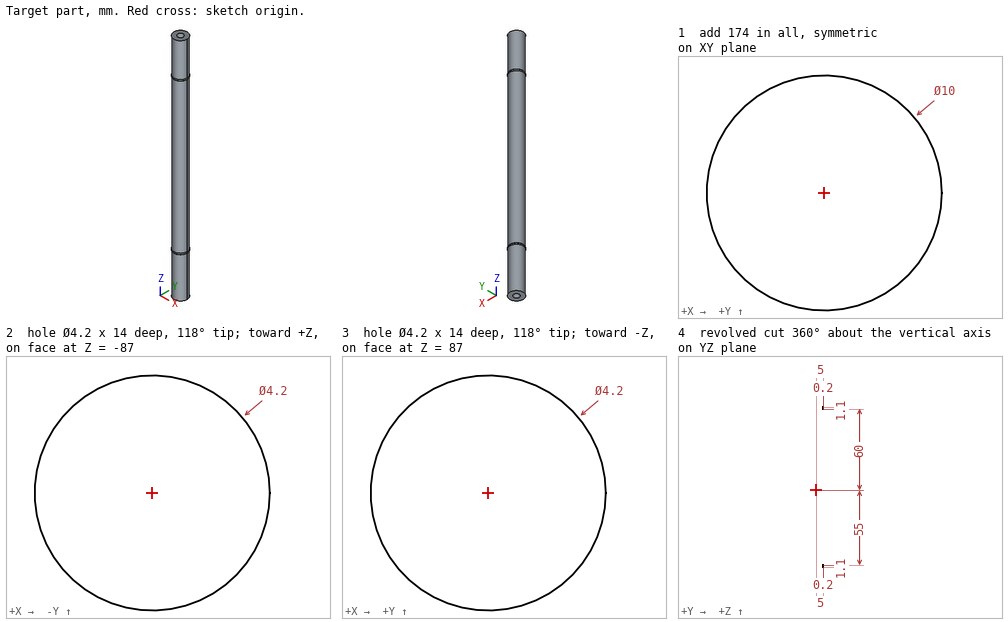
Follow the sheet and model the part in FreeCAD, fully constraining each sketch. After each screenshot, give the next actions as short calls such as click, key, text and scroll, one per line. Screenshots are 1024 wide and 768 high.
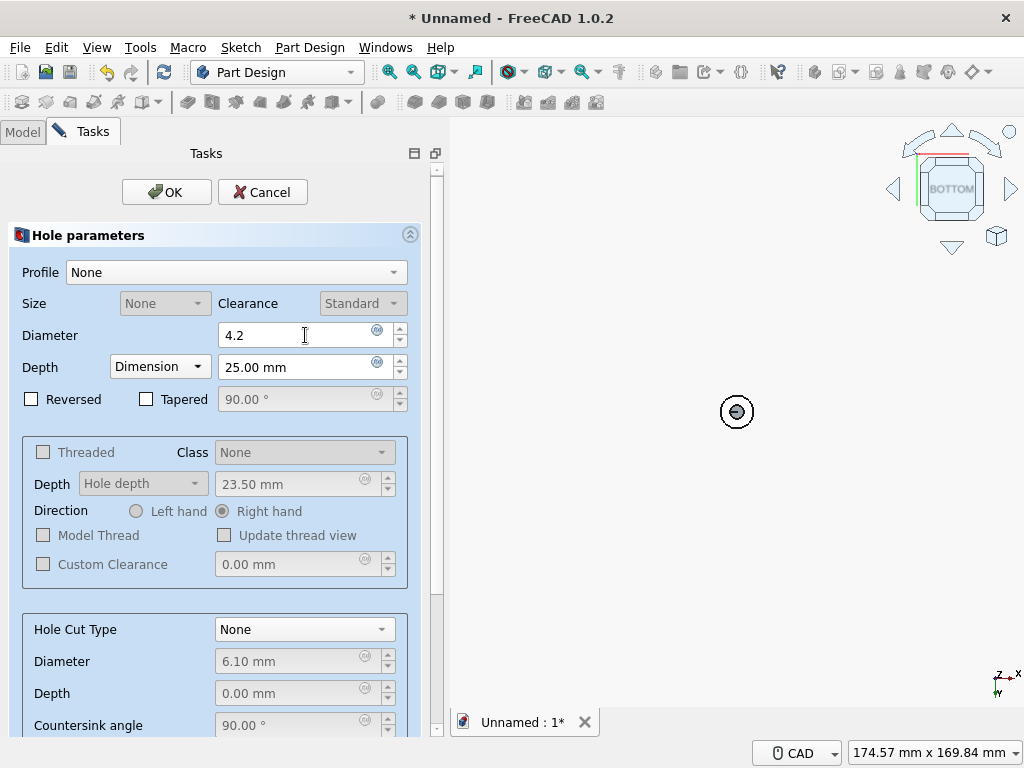
triple_click(305, 367)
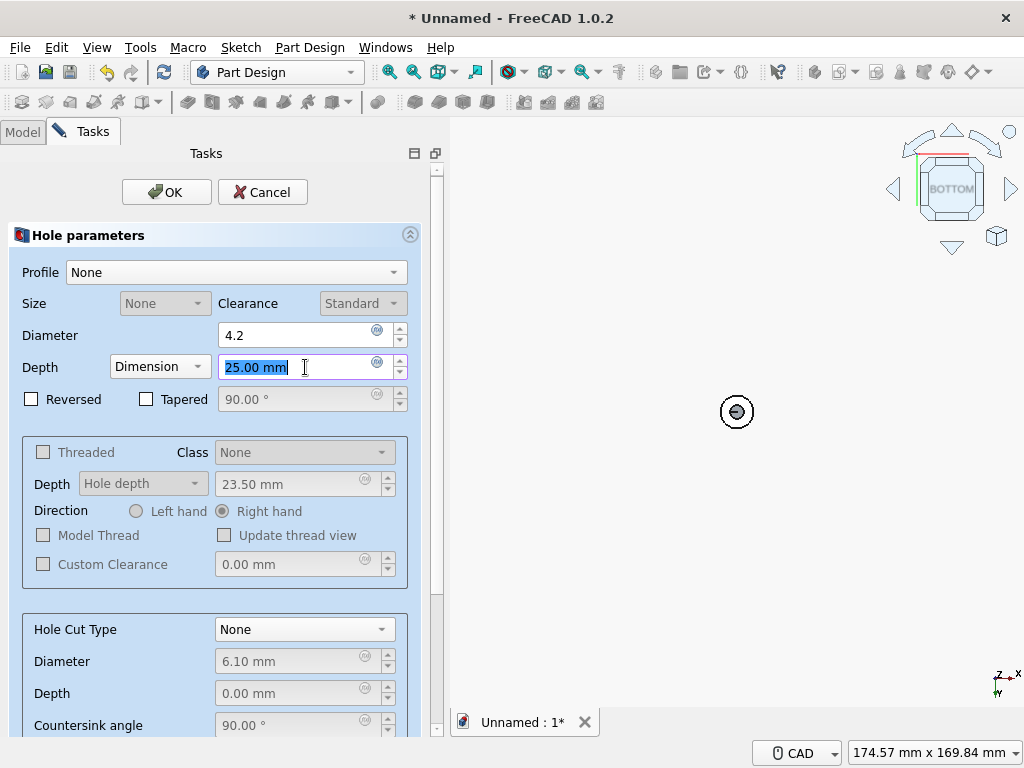
text(14)
key(Tab)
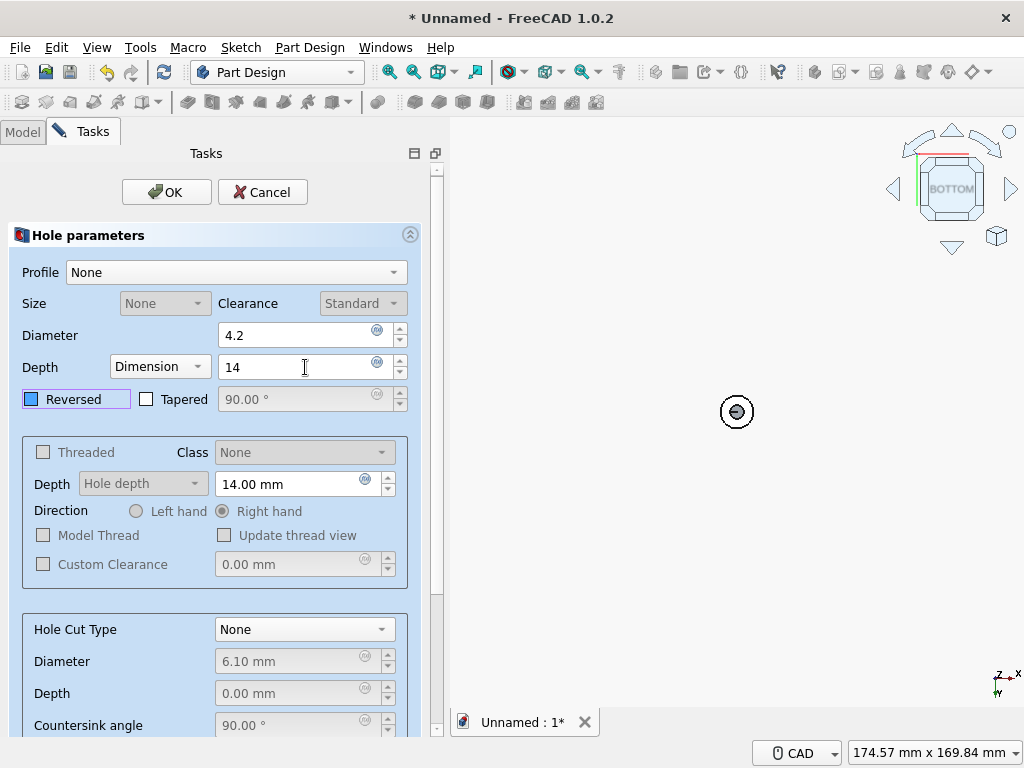
click(167, 192)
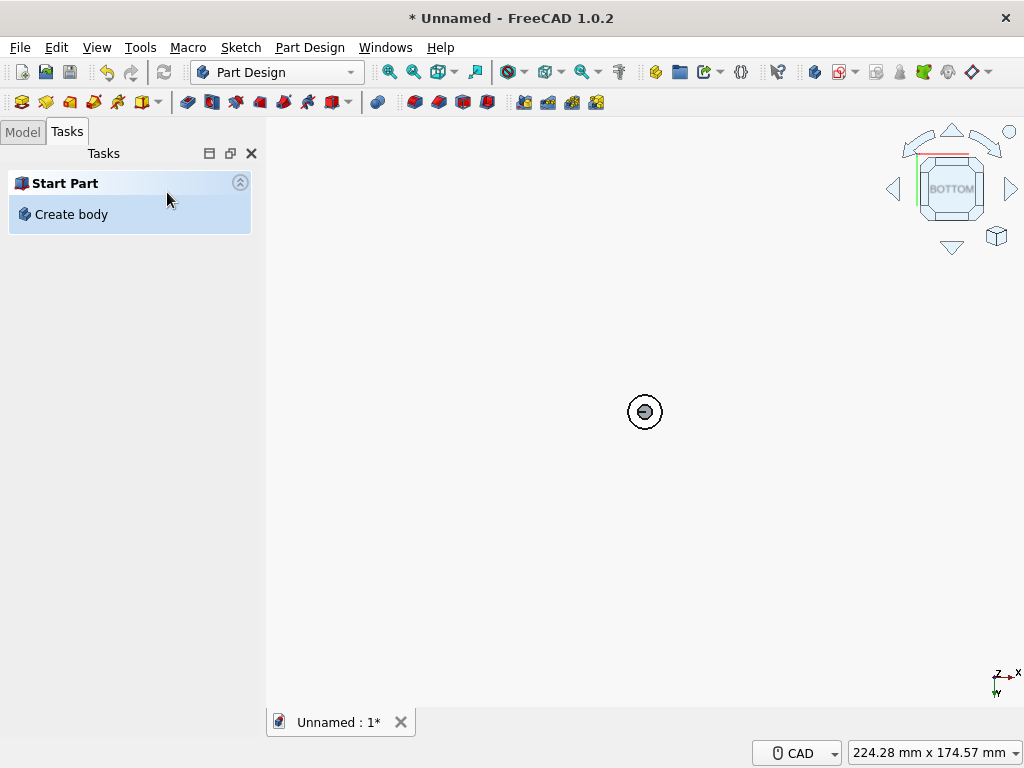
click(390, 72)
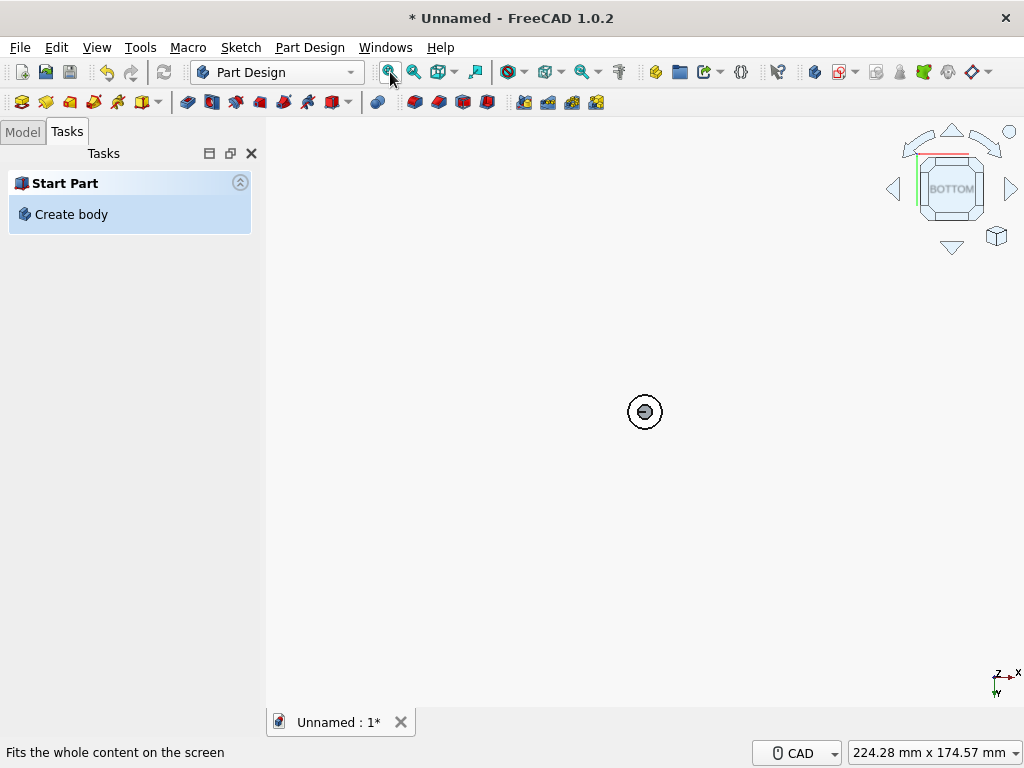
key(0)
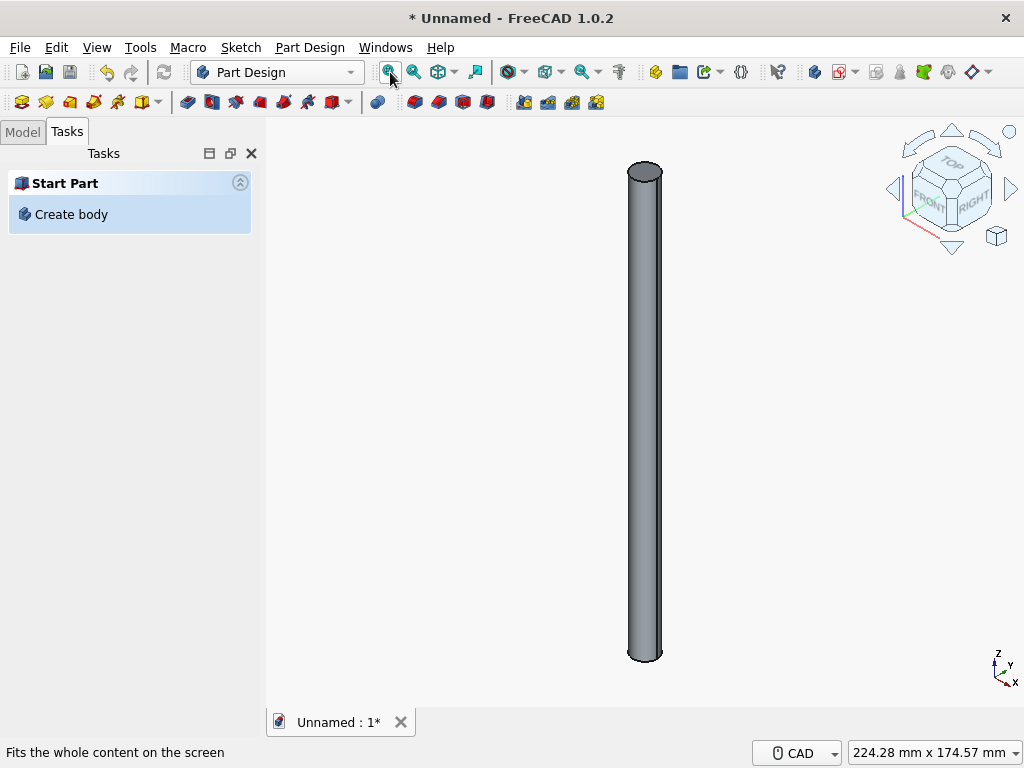
click(645, 171)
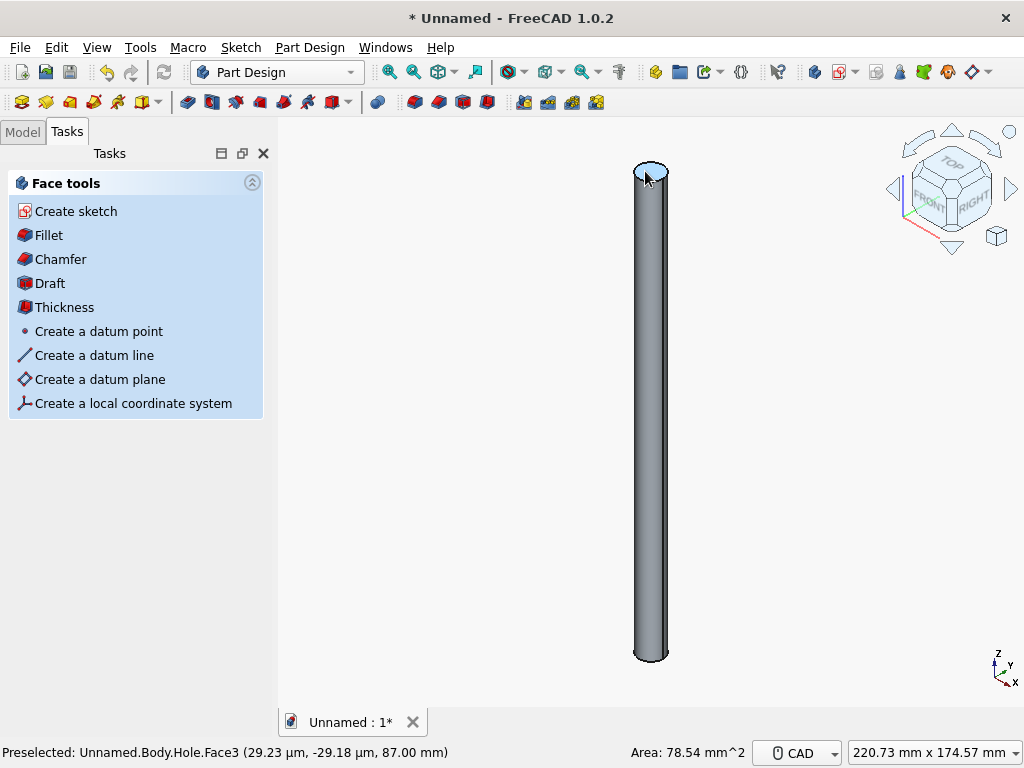
click(840, 72)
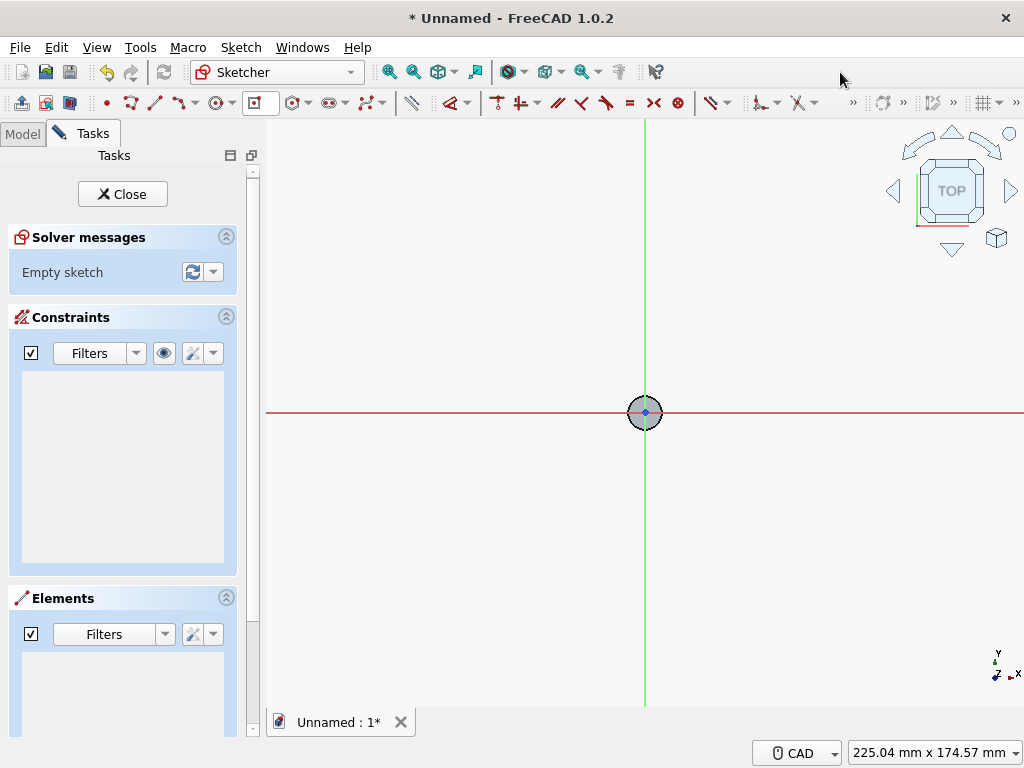
scroll(649, 413, up, 15)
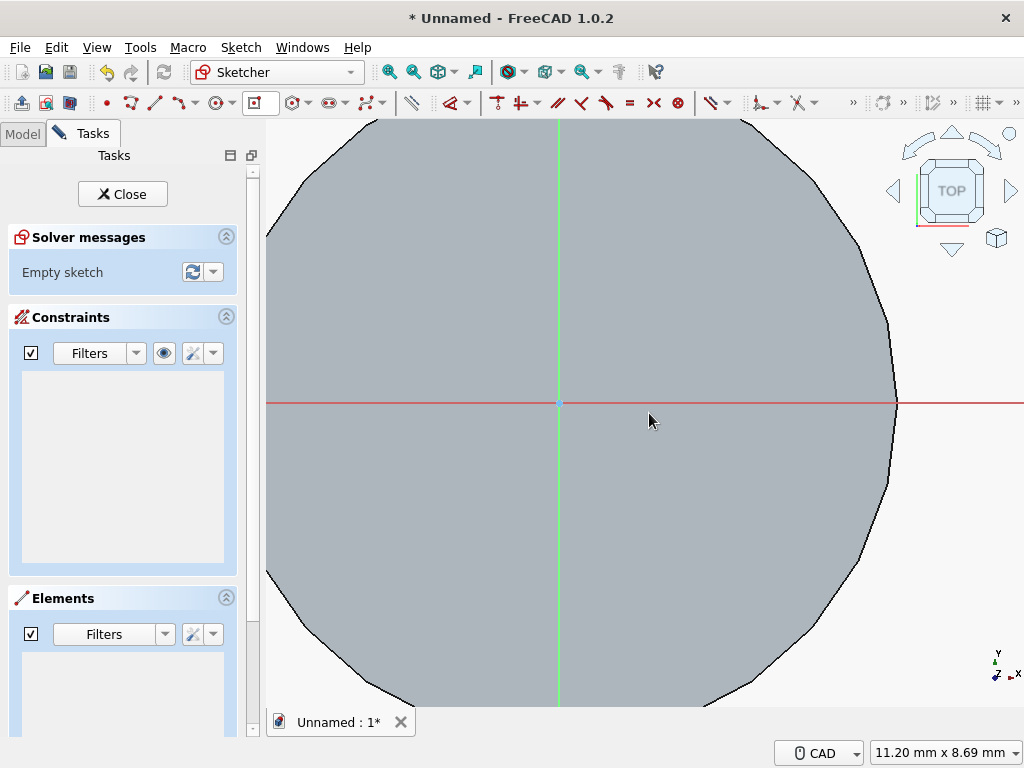
click(216, 104)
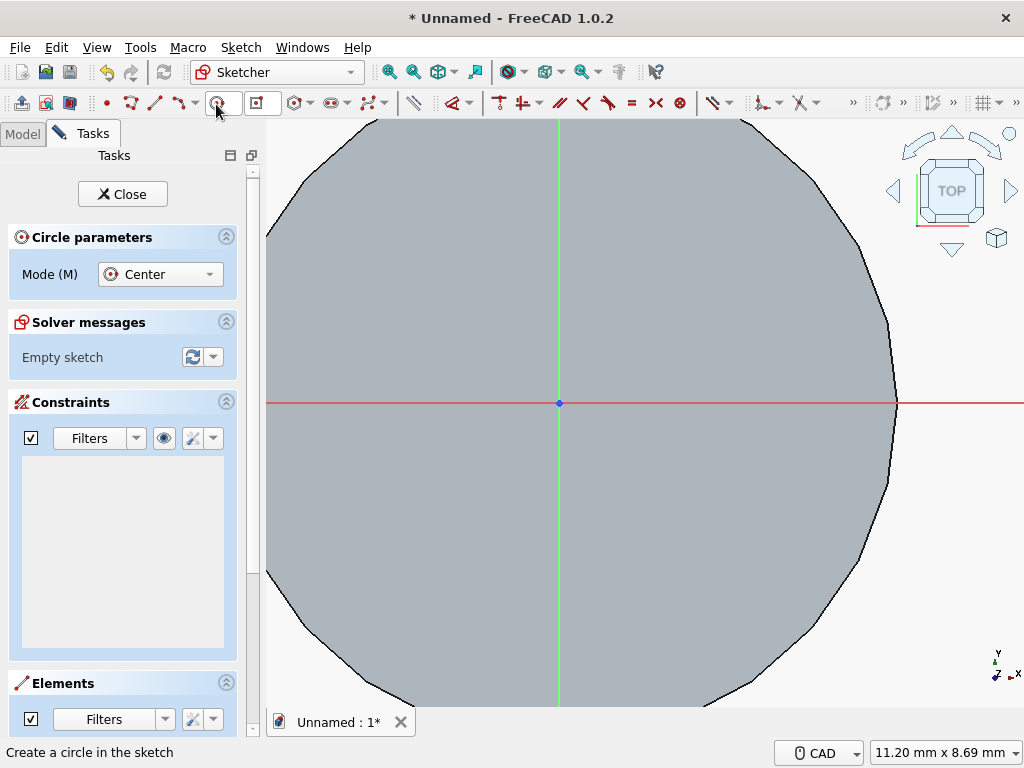
click(559, 403)
move(659, 303)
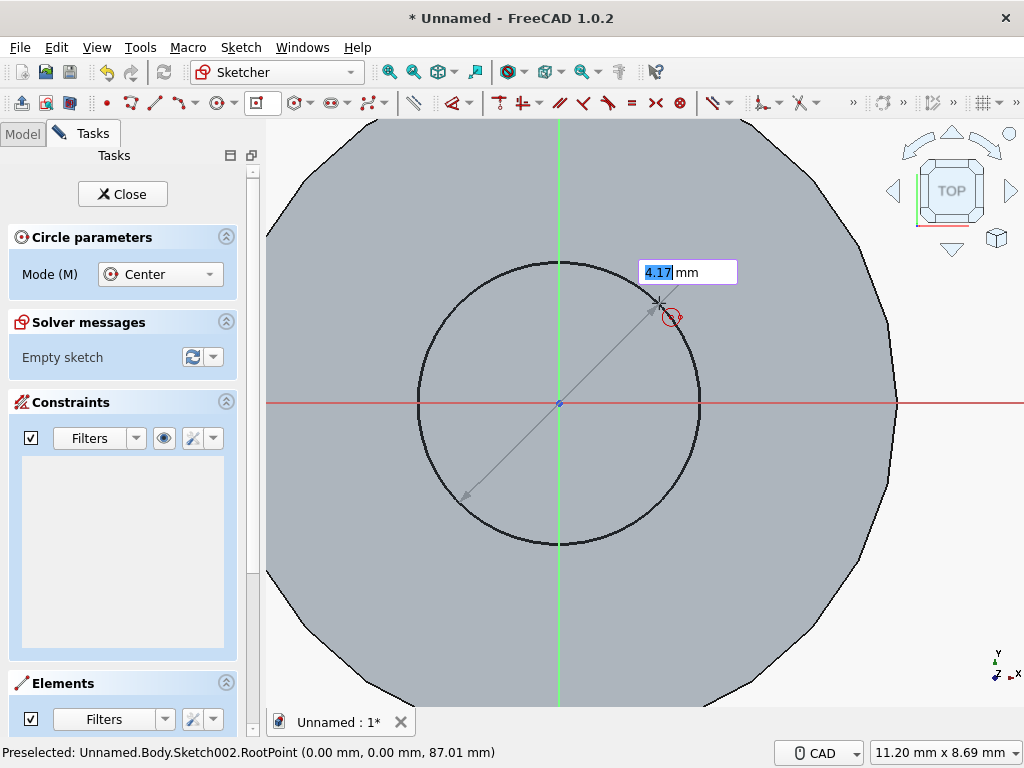
text(4.2)
key(Return)
key(Escape)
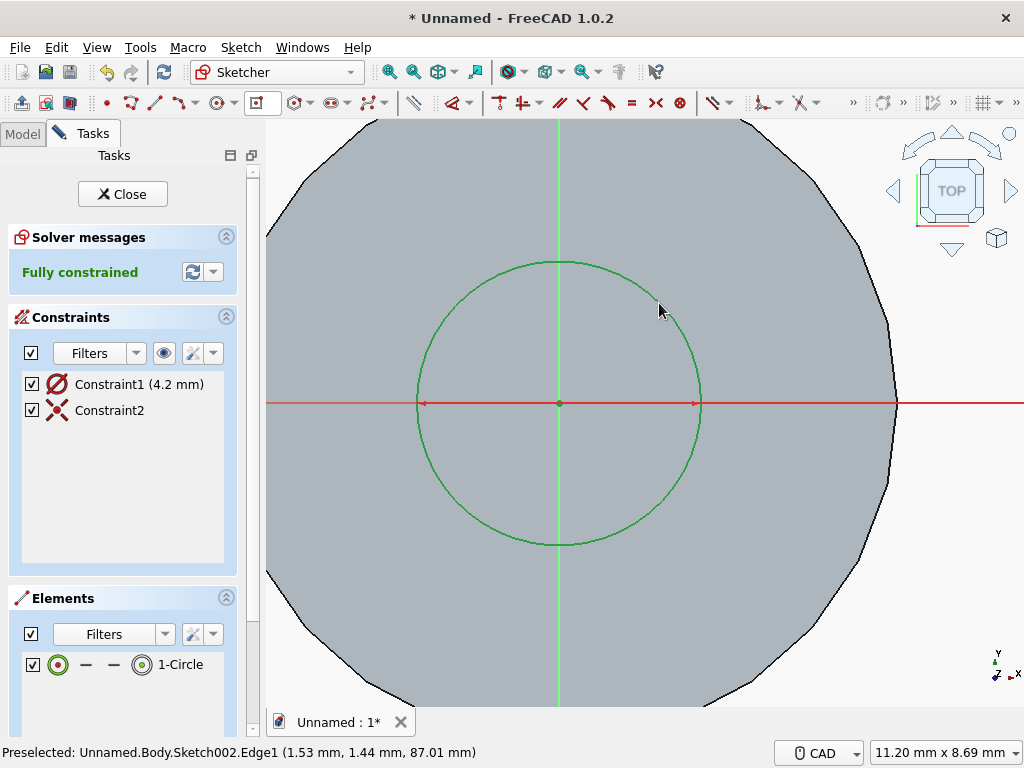
click(123, 194)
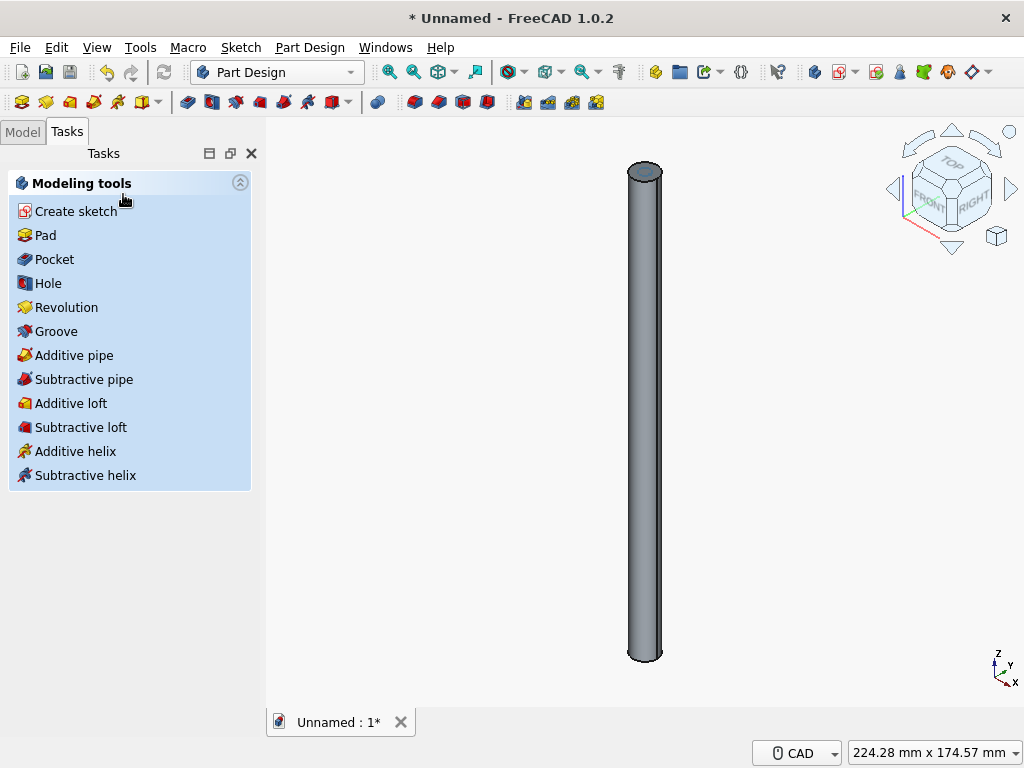
click(212, 102)